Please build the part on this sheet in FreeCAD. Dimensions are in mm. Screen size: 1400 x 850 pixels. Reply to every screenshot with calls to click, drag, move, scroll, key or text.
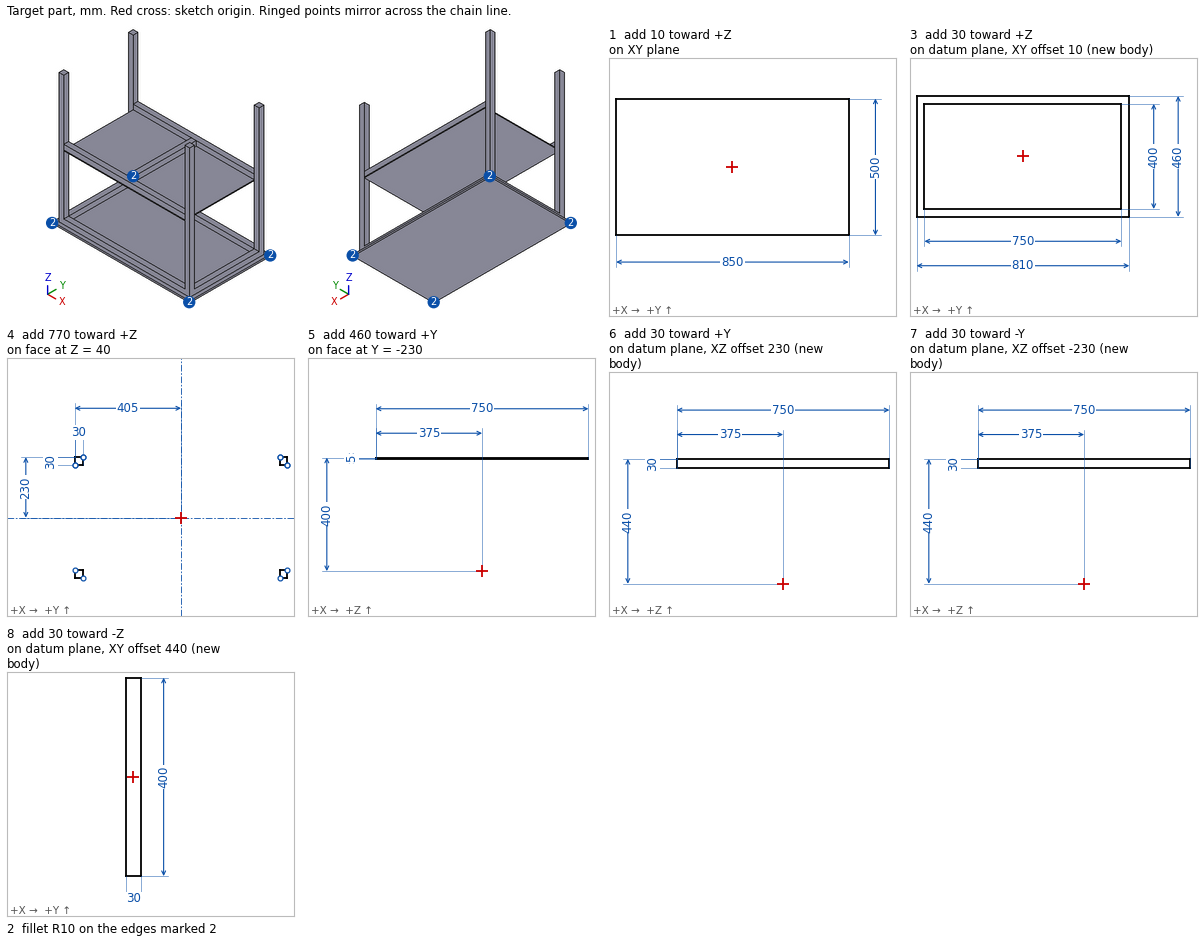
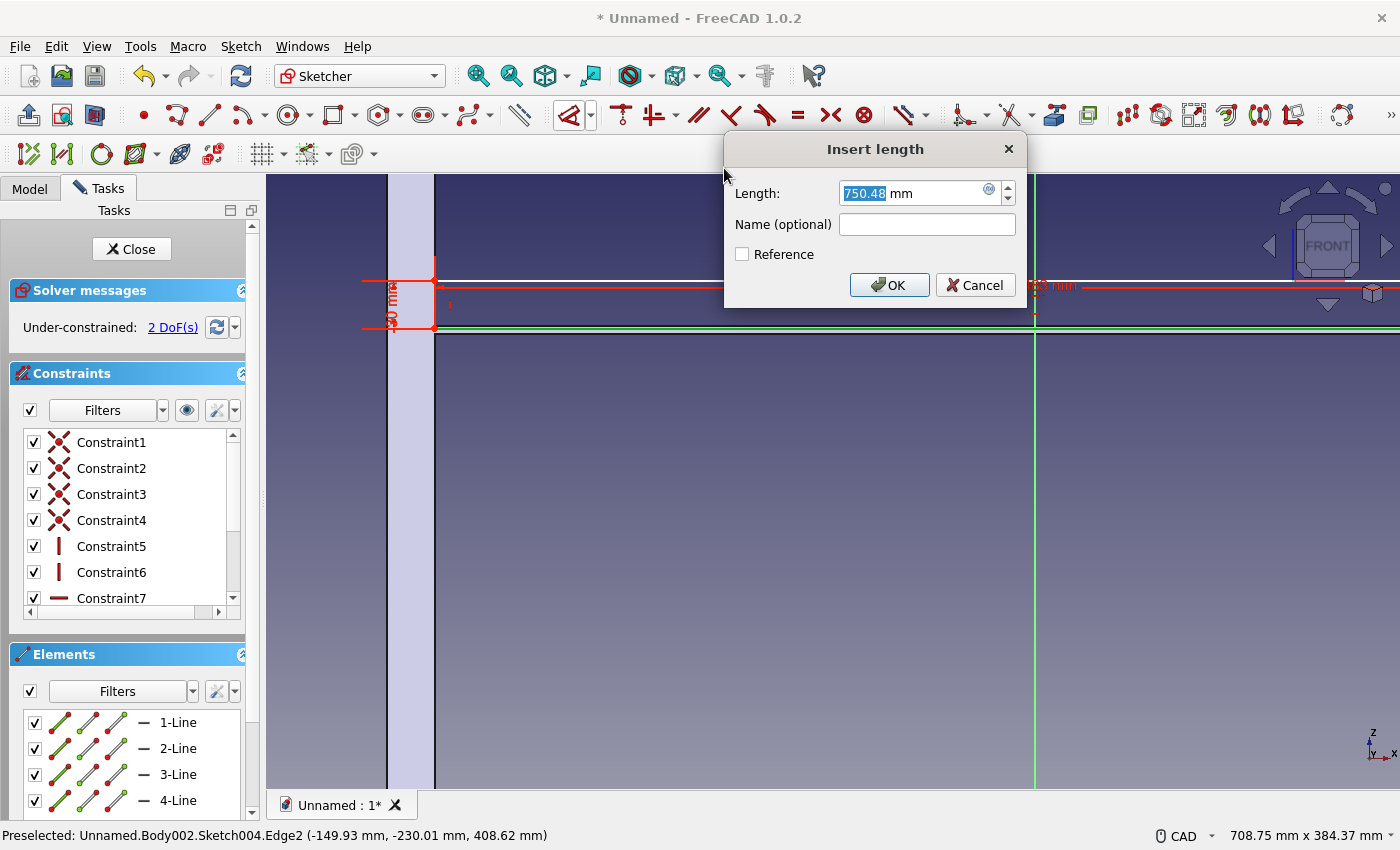
text(750)
key(Return)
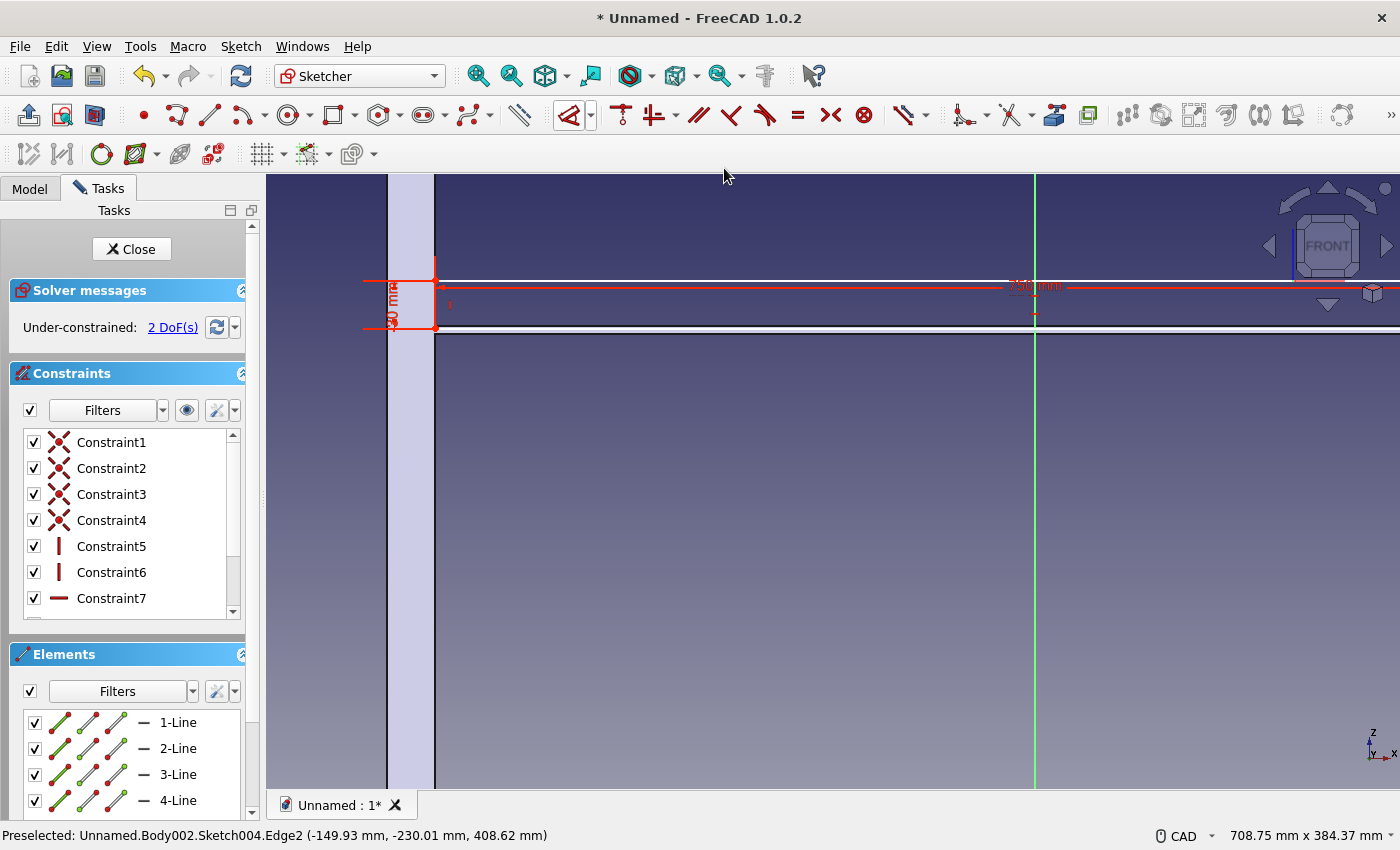
click(435, 280)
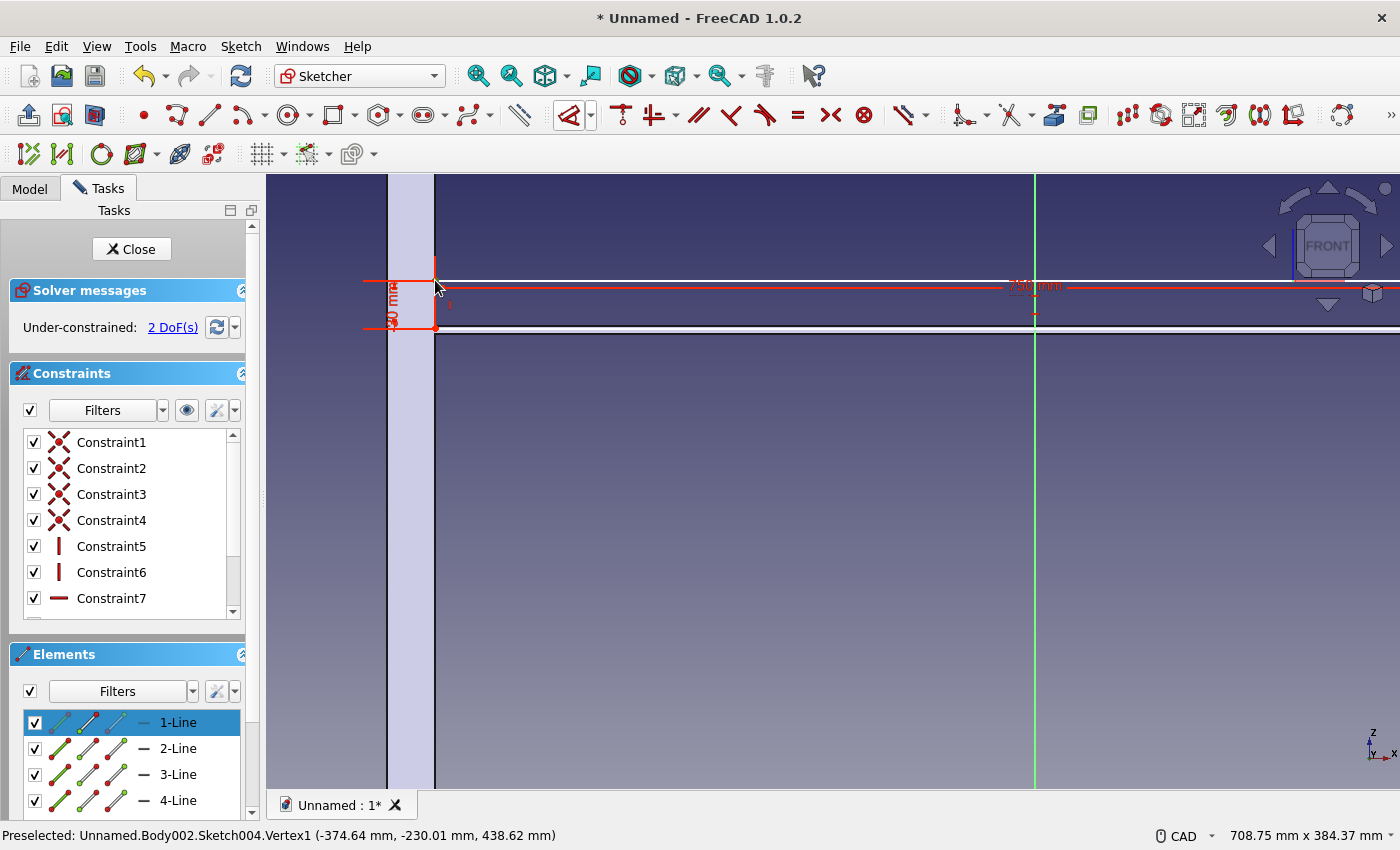
click(590, 116)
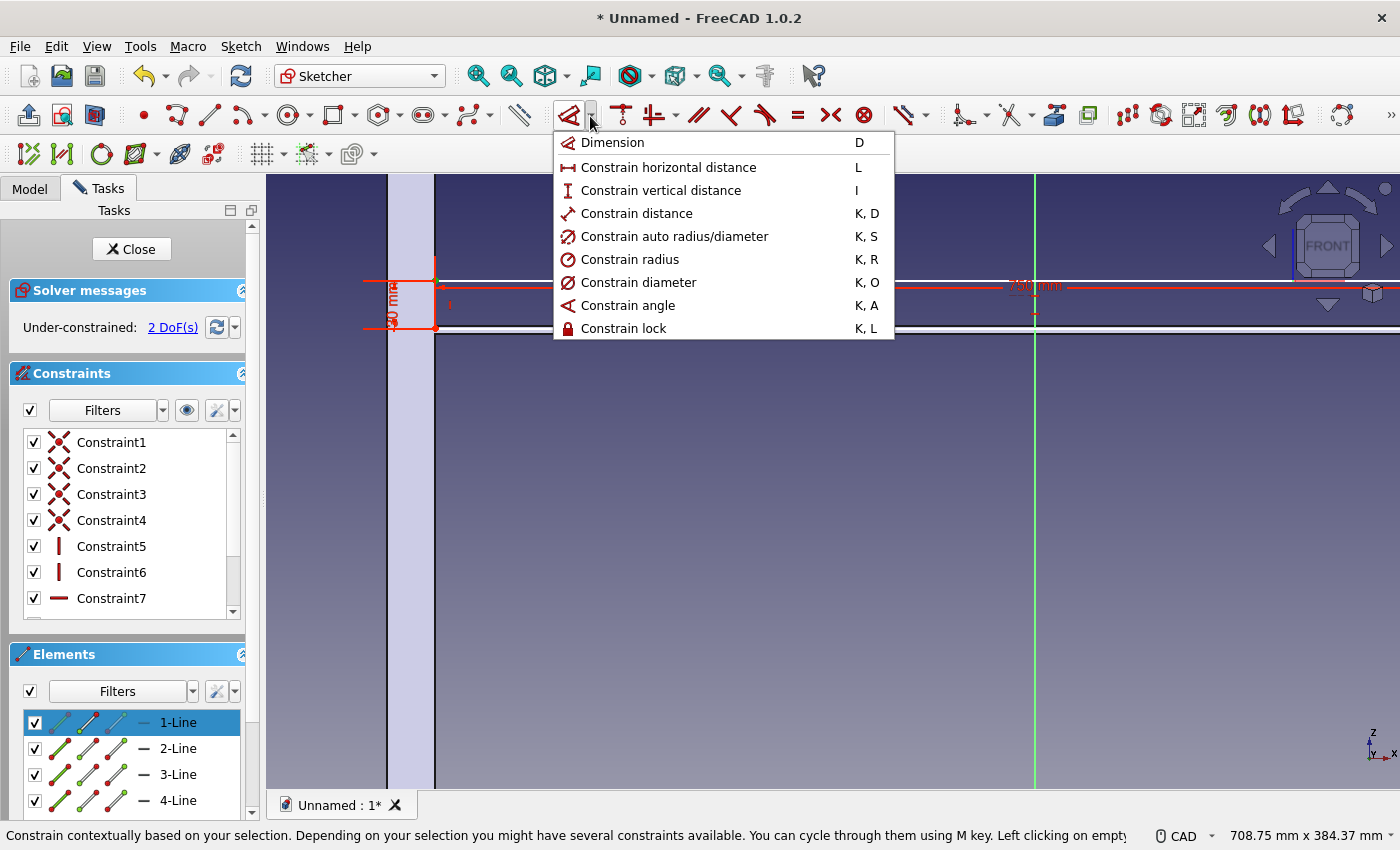
click(724, 168)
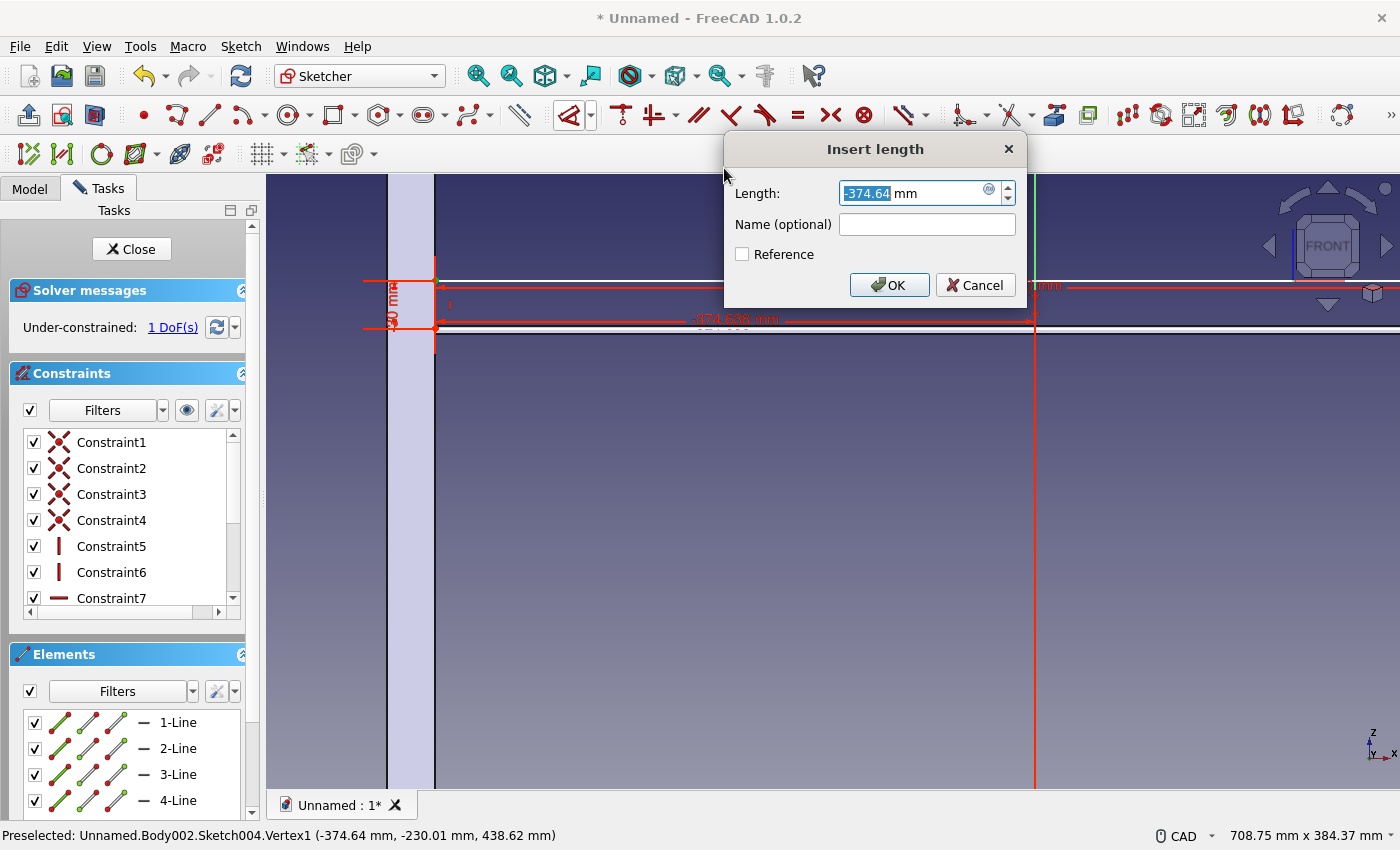
text(-375)
key(Return)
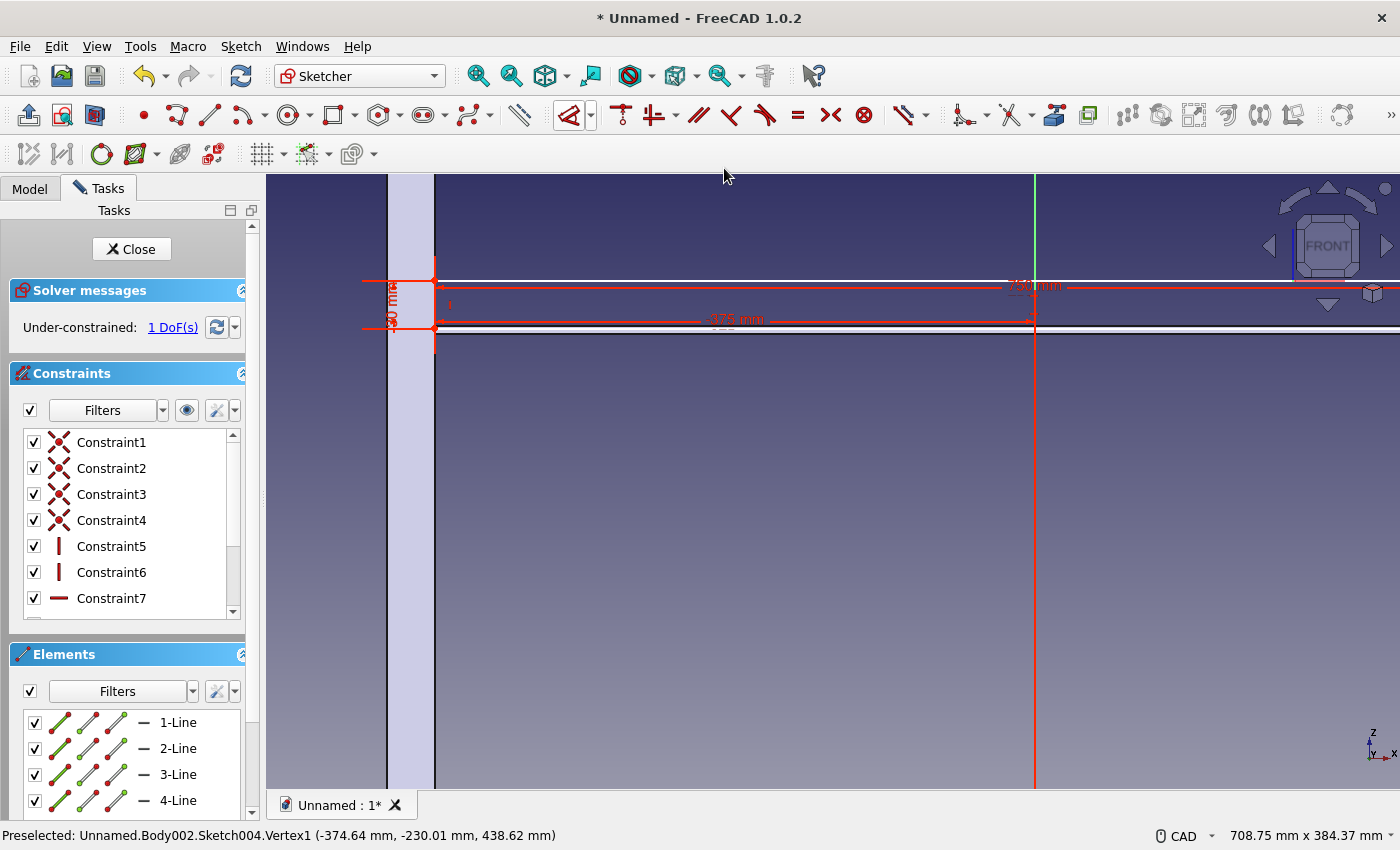
click(435, 280)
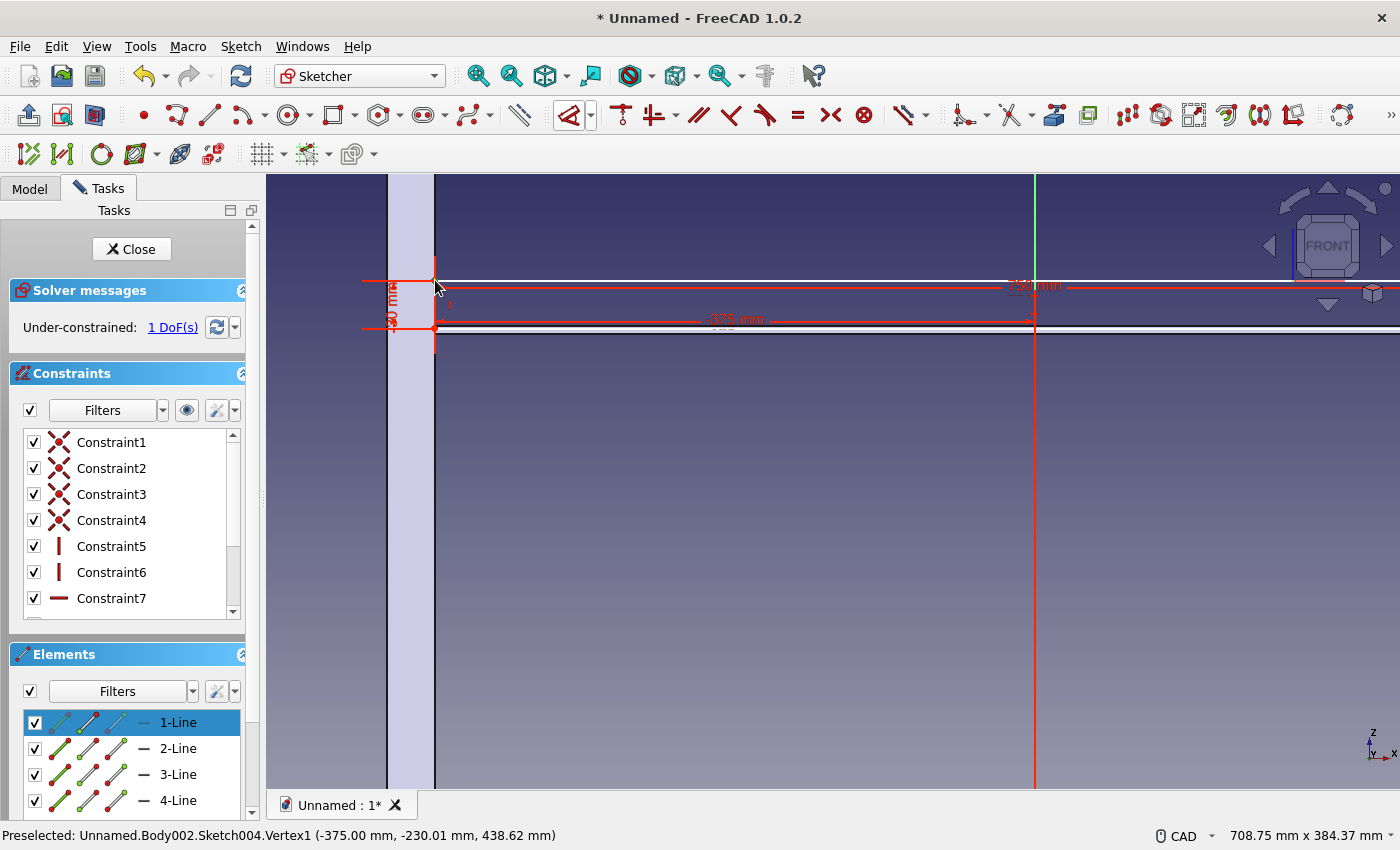
click(590, 116)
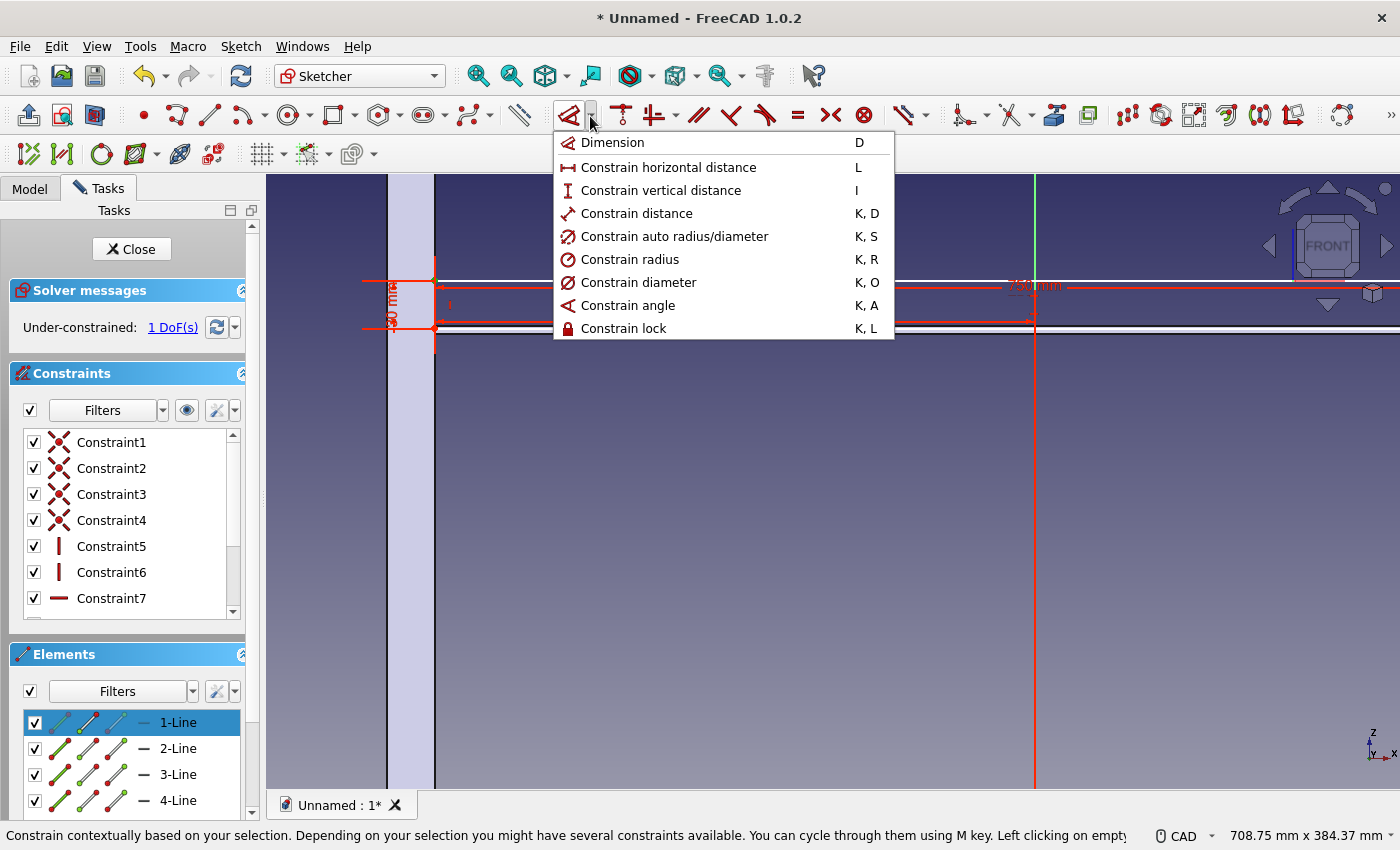
click(724, 190)